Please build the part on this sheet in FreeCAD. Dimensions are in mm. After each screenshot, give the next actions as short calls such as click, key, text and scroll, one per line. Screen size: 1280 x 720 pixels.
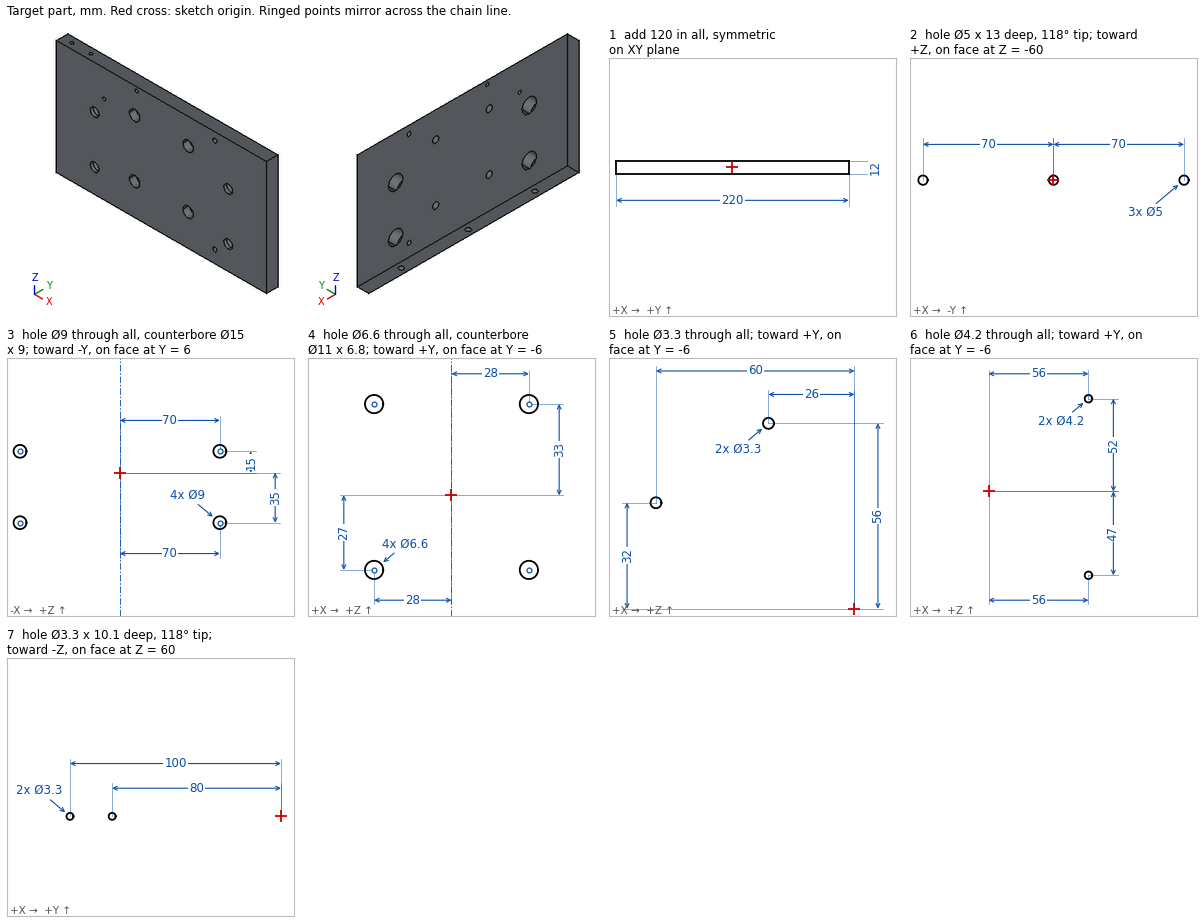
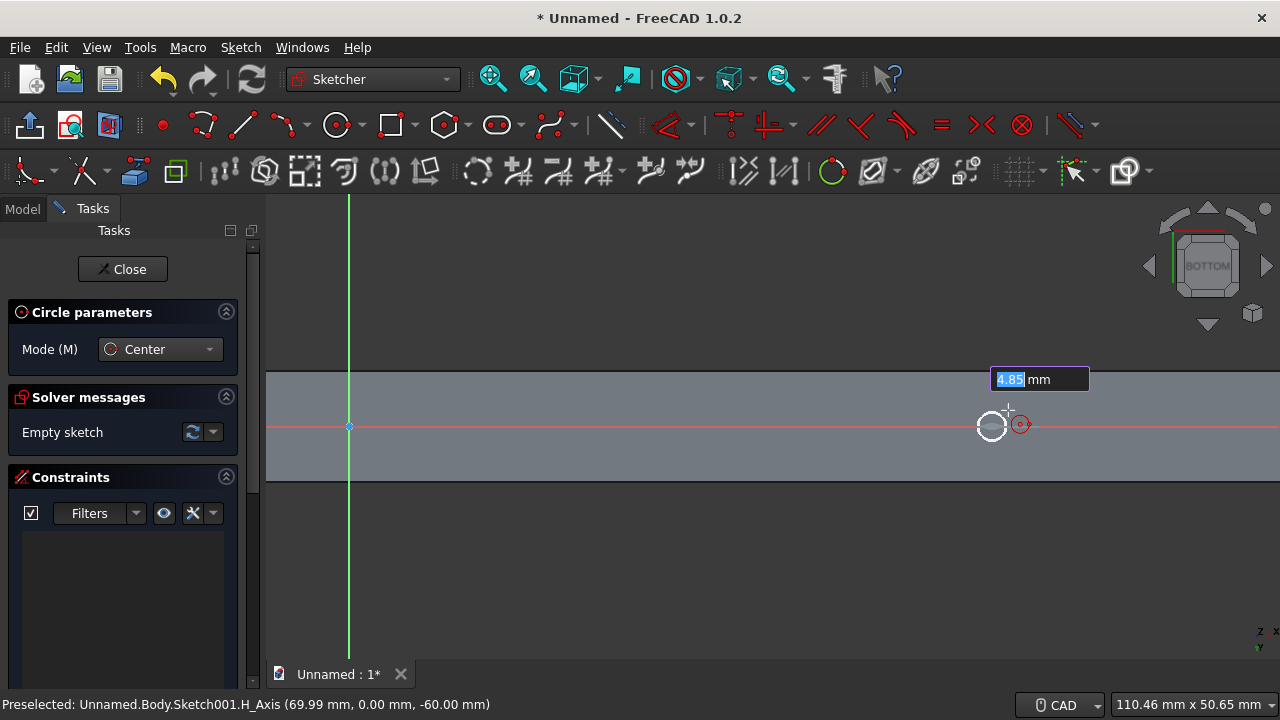
text(5)
key(Return)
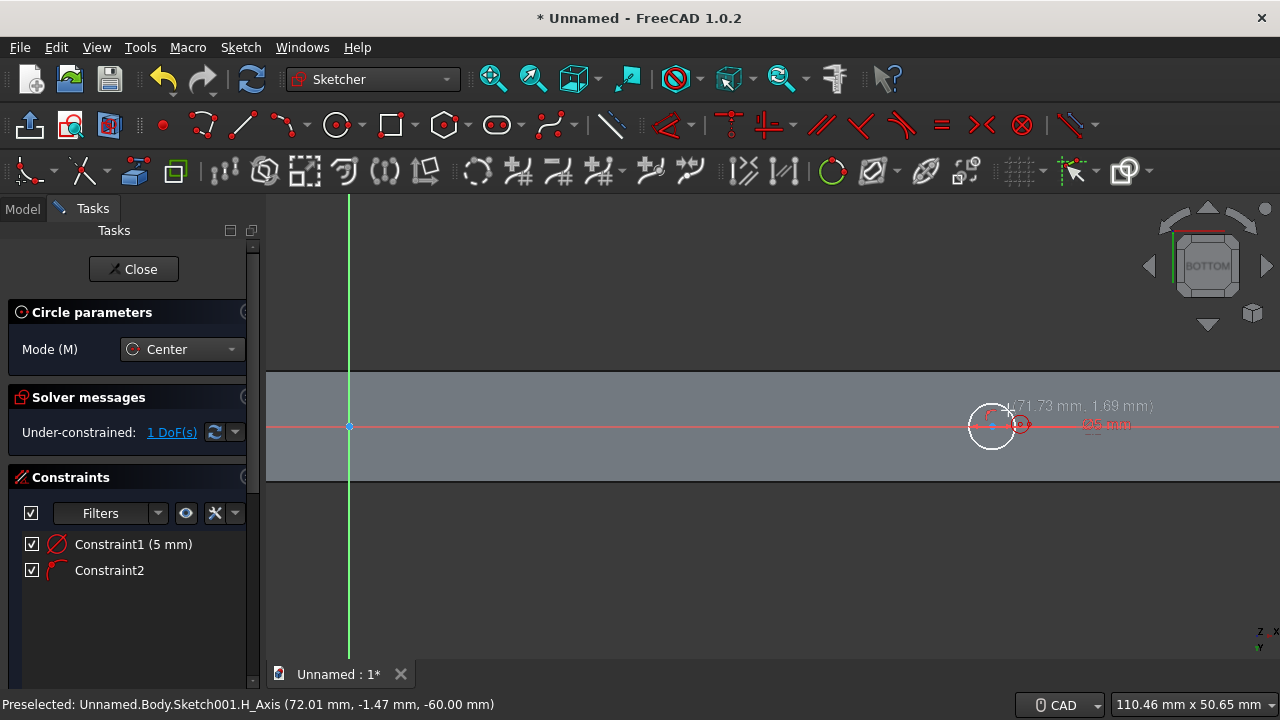
click(349, 426)
move(366, 410)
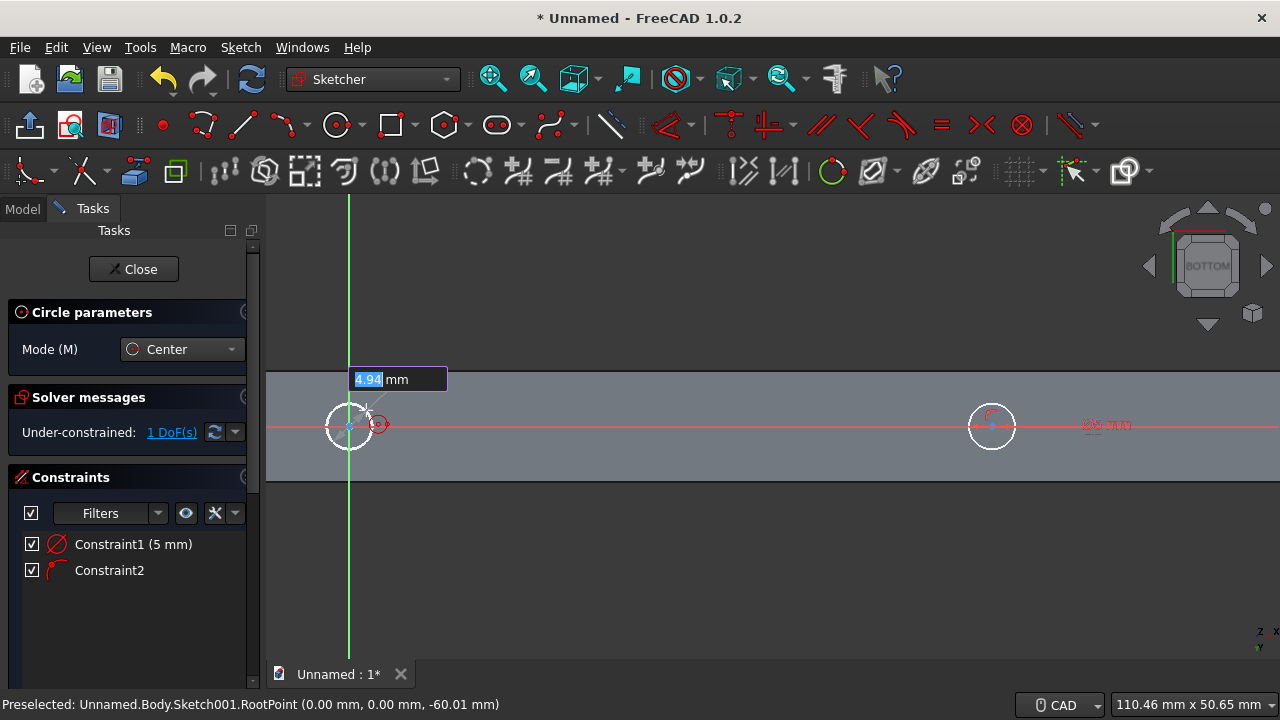
text(5)
key(Return)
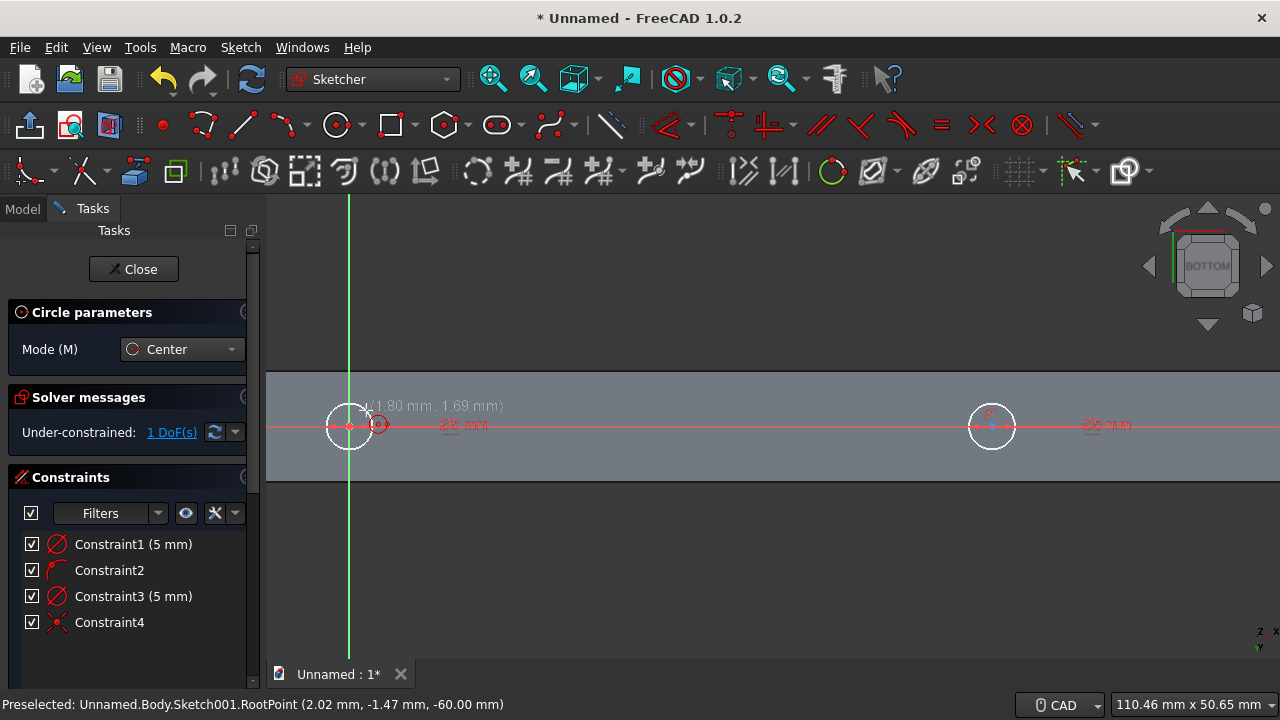
scroll(994, 426, down, 4)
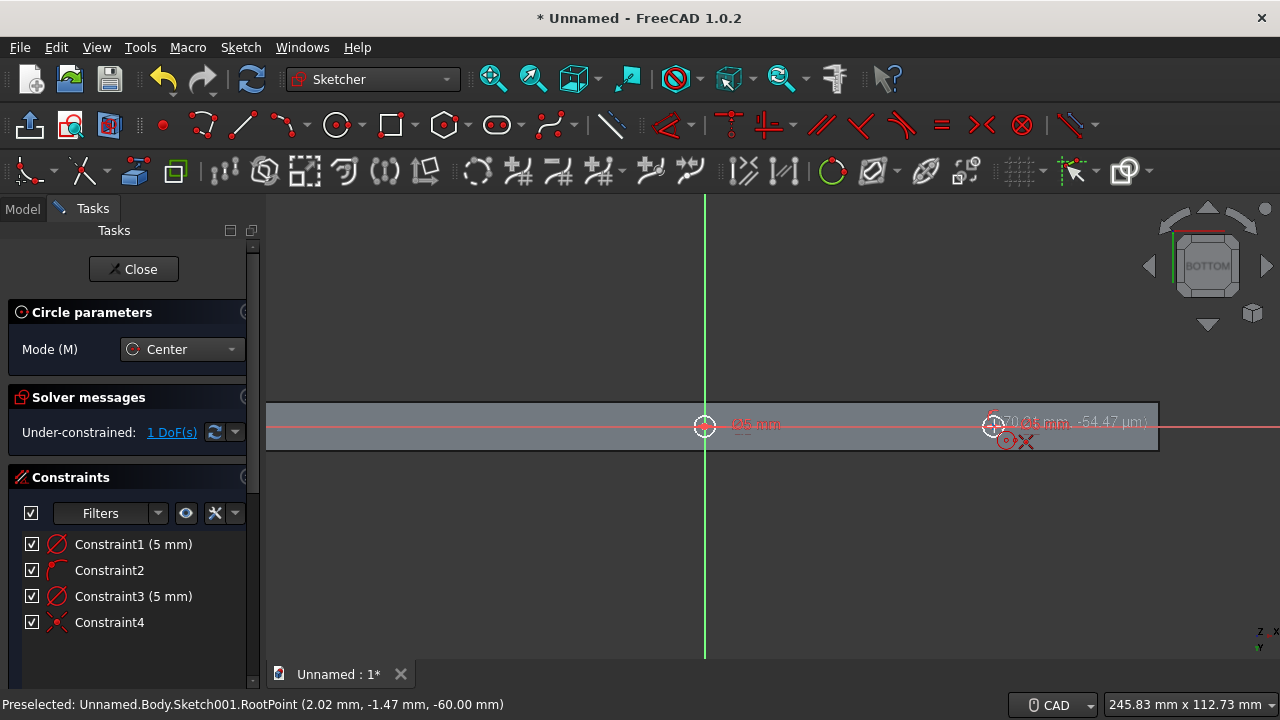
scroll(416, 426, up, 4)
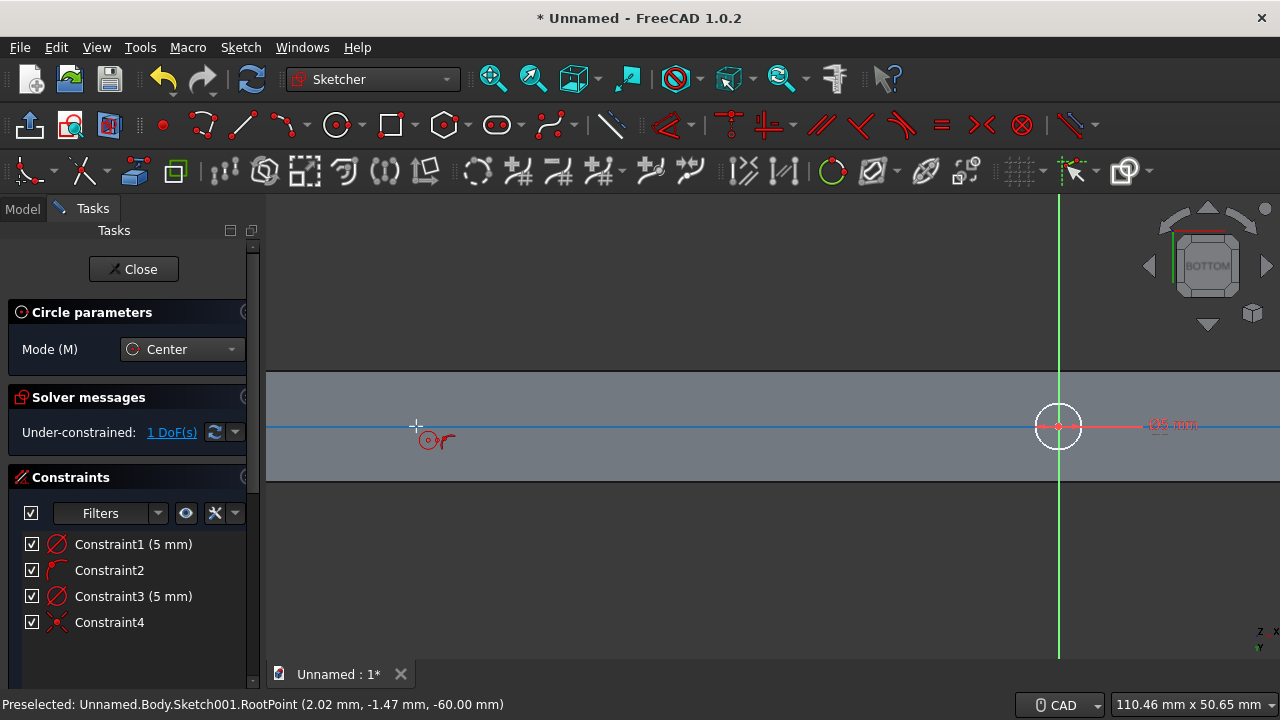
click(416, 426)
move(432, 410)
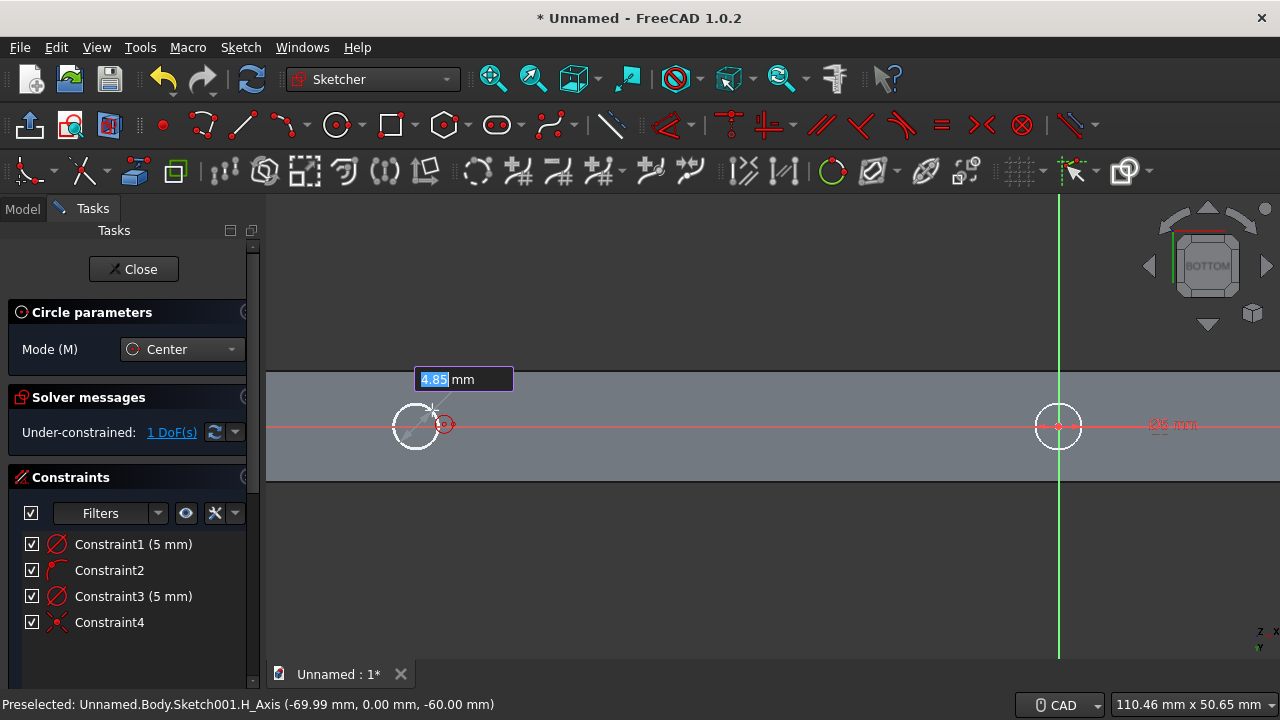
text(5)
key(Return)
key(Escape)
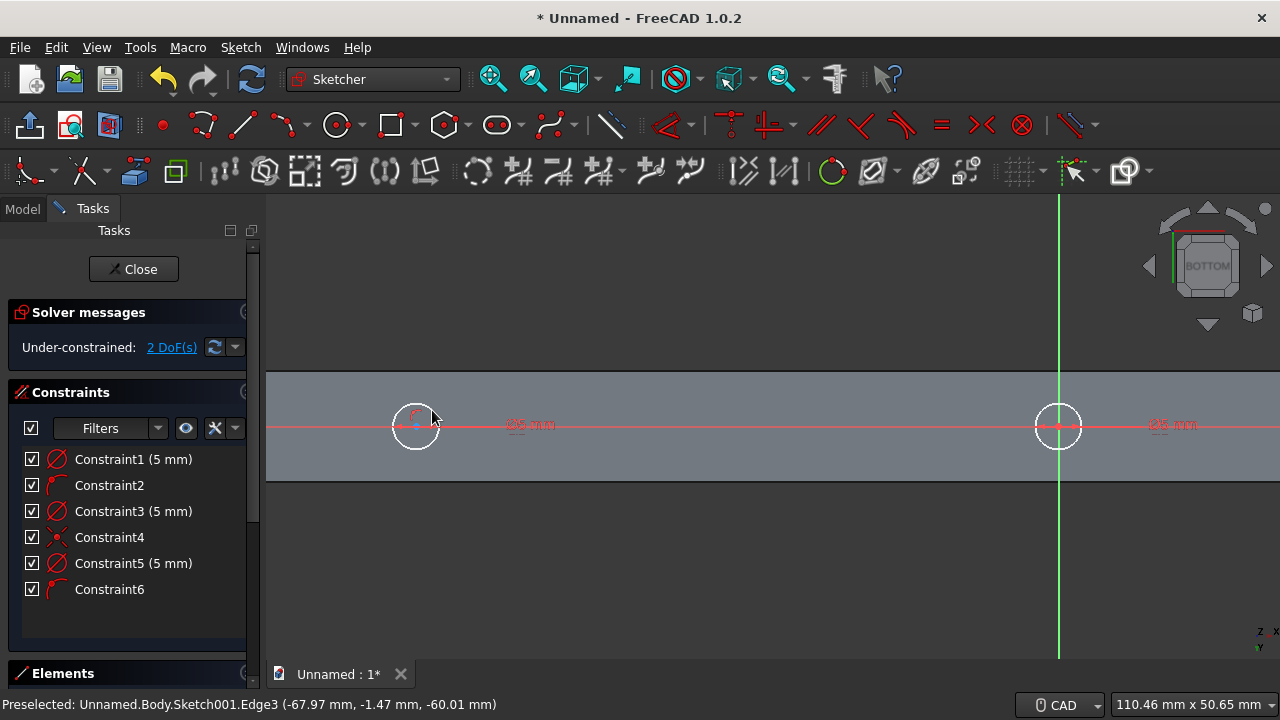
click(666, 126)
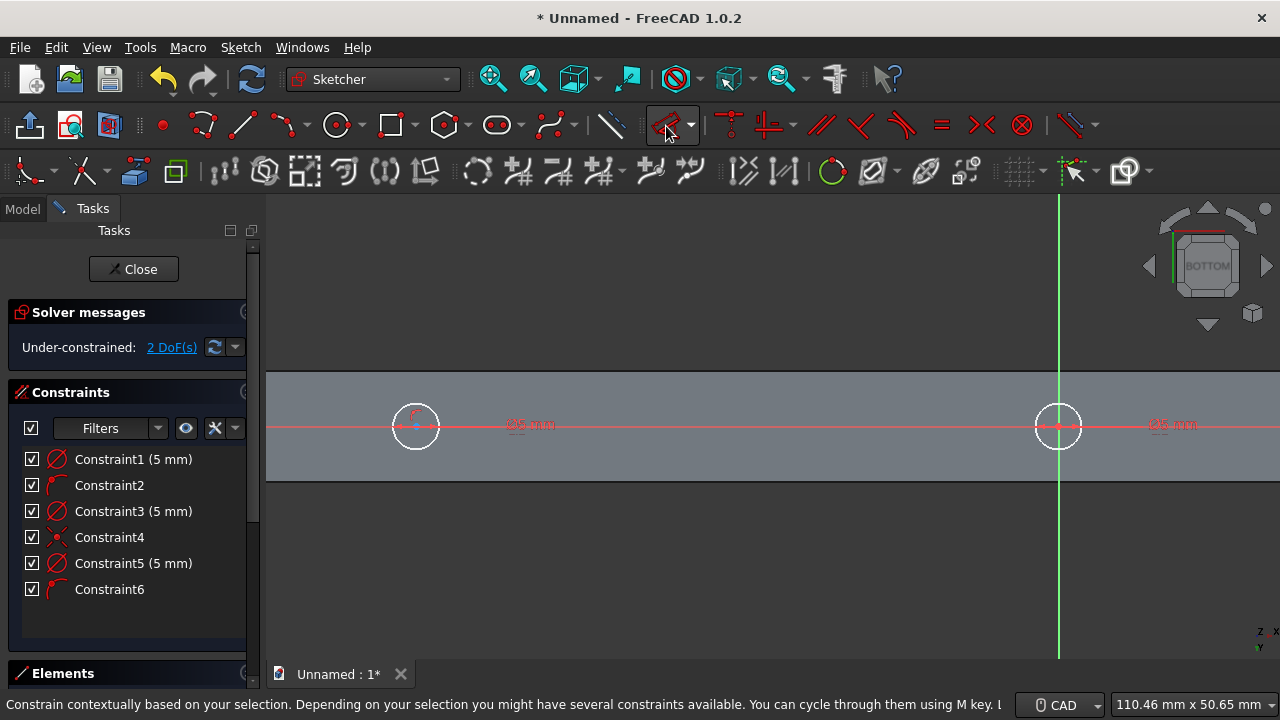
scroll(416, 426, down, 4)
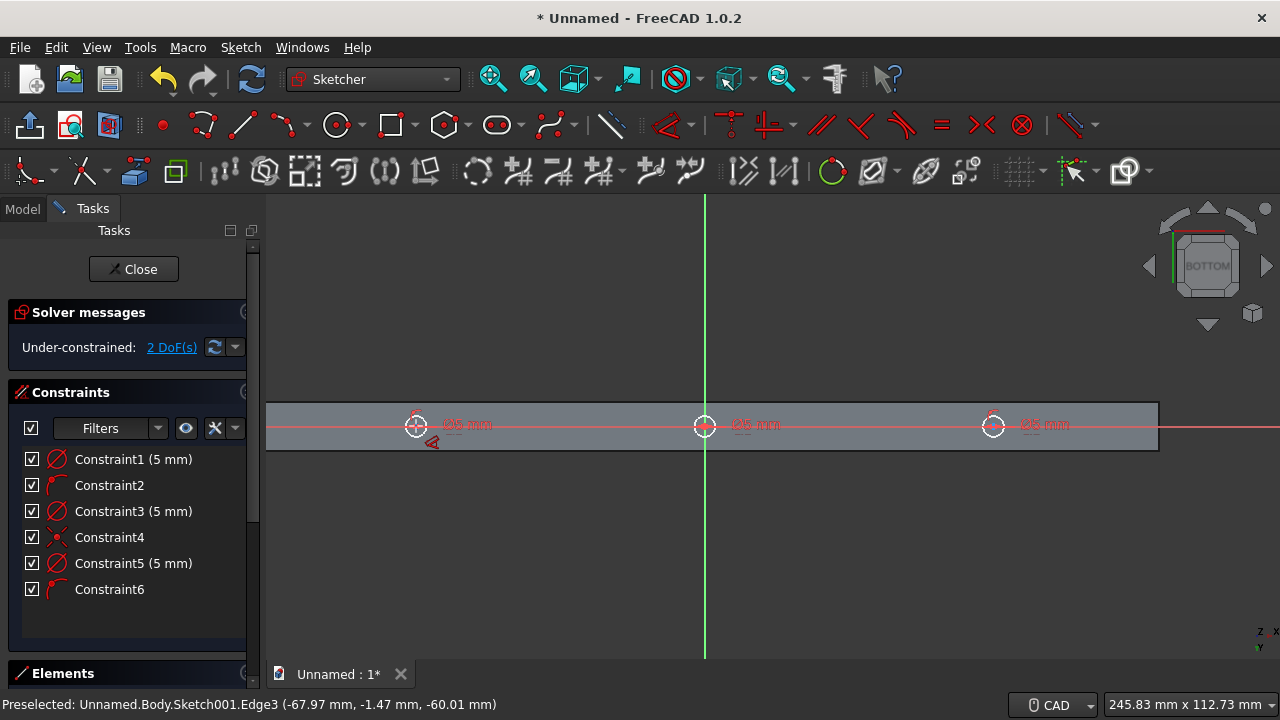
click(993, 426)
click(849, 460)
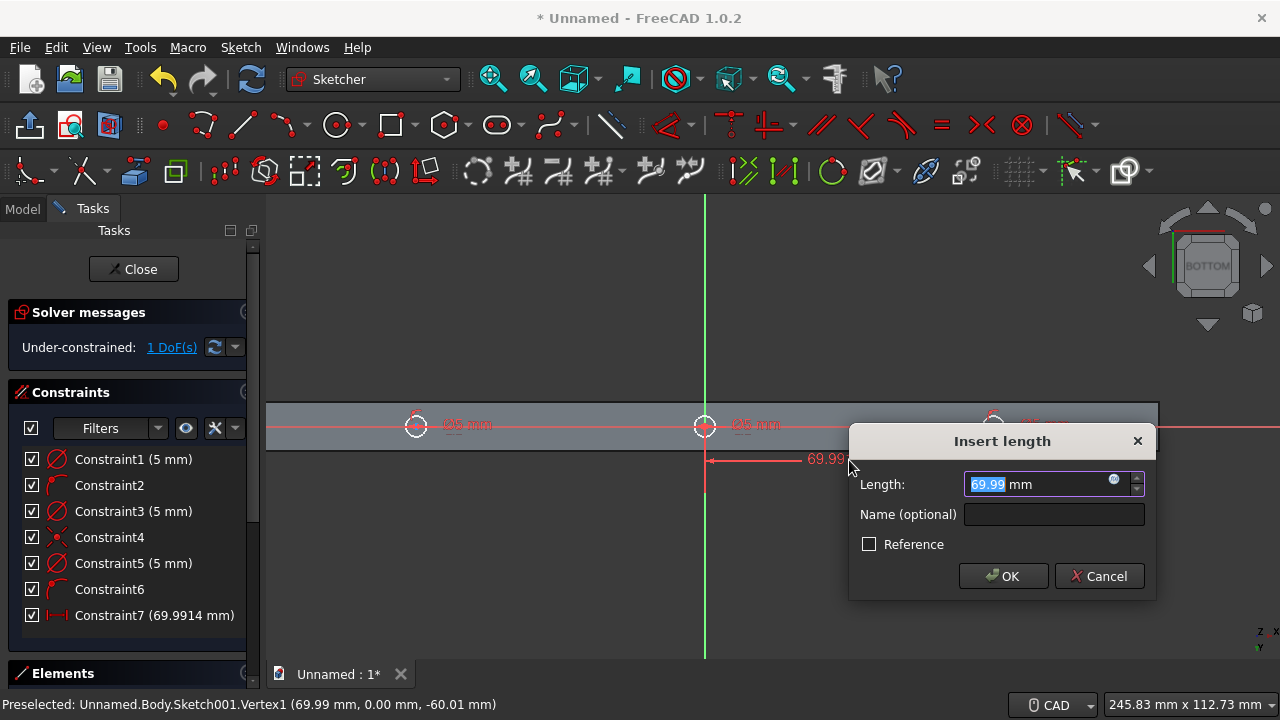
text(70)
key(Return)